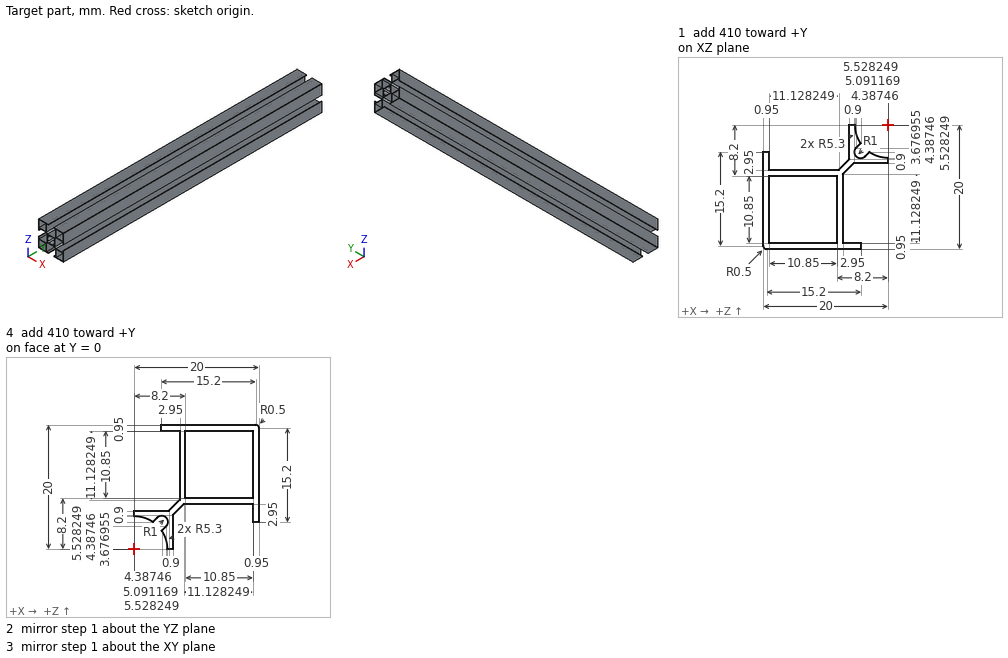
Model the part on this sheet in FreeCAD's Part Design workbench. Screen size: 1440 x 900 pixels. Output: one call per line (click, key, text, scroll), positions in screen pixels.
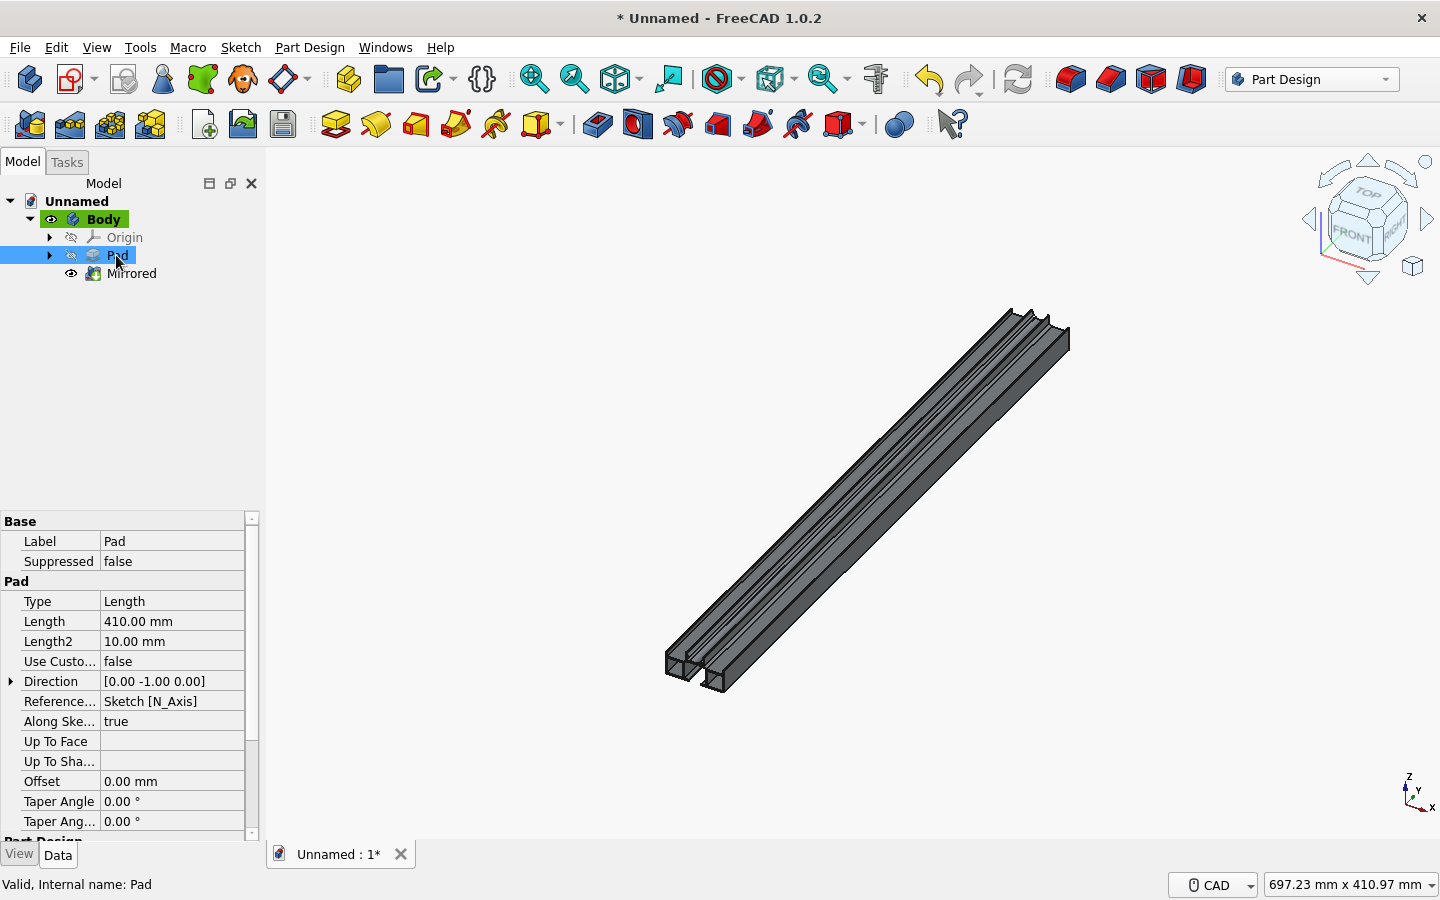
click(30, 124)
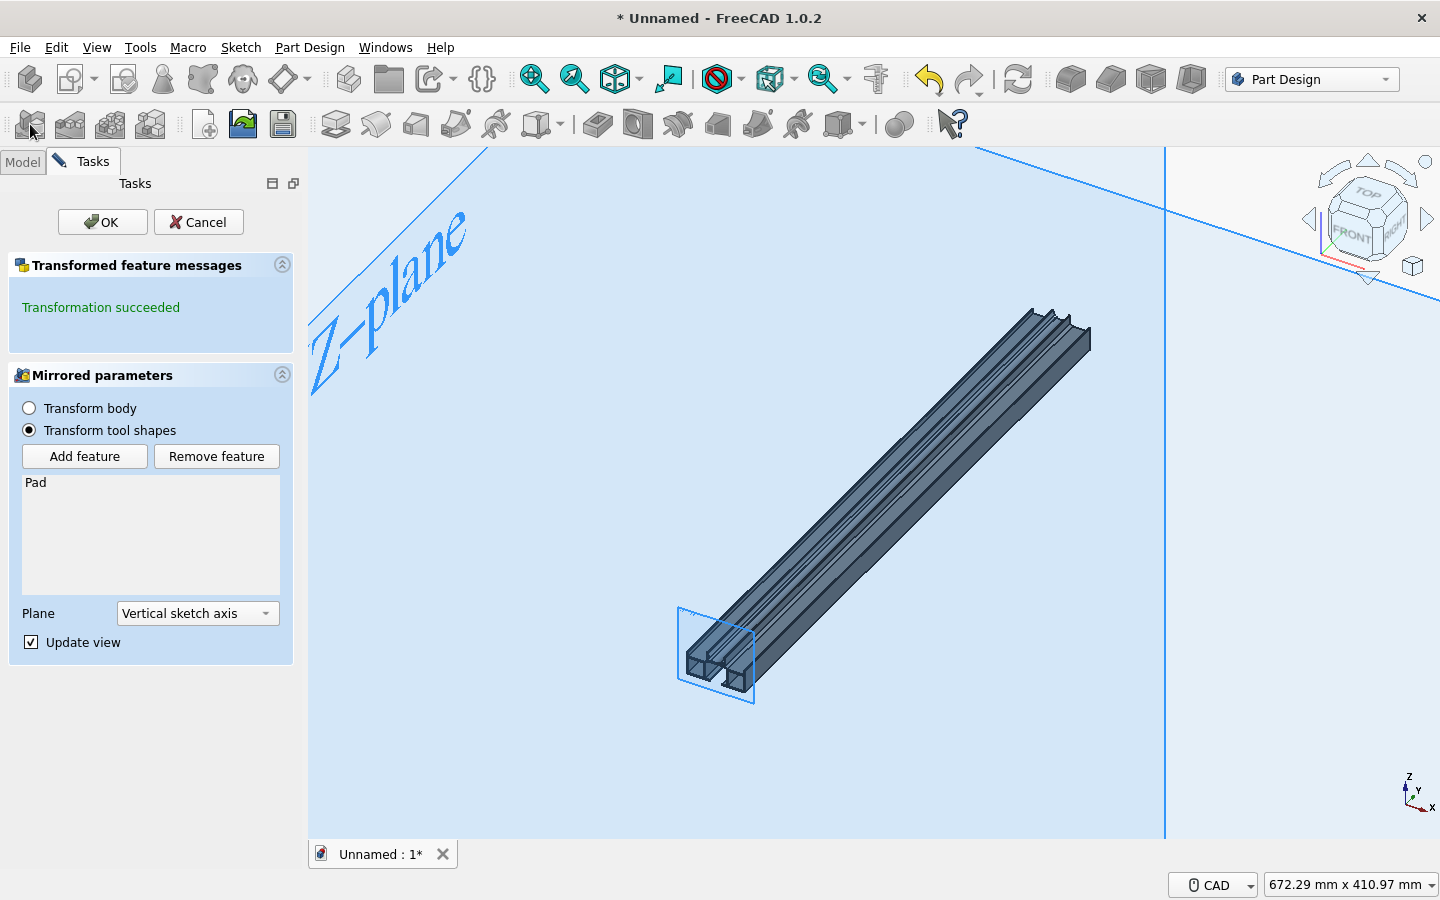
click(198, 614)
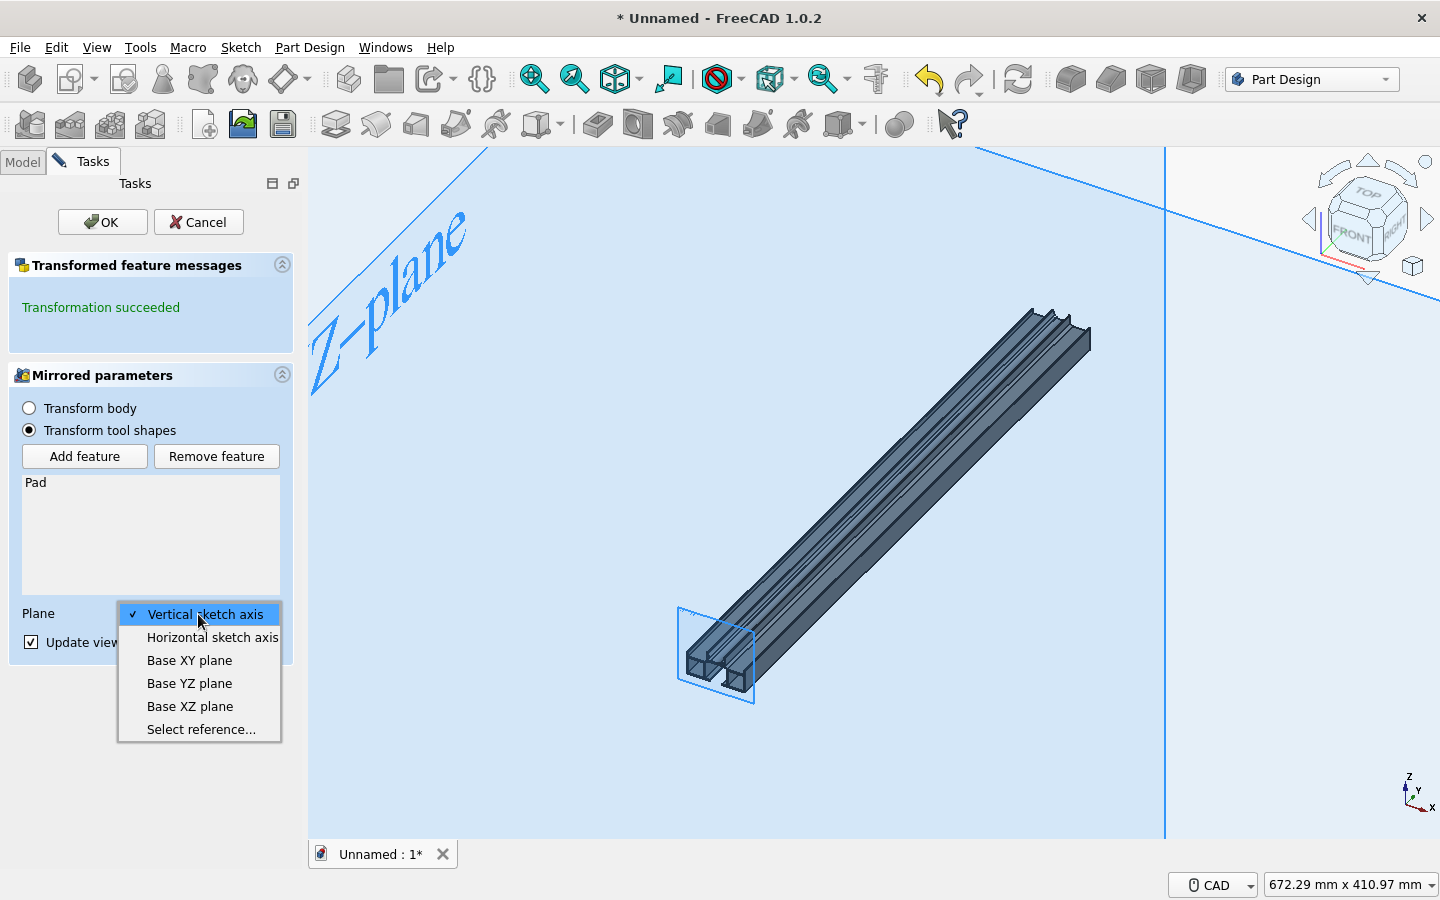
click(198, 660)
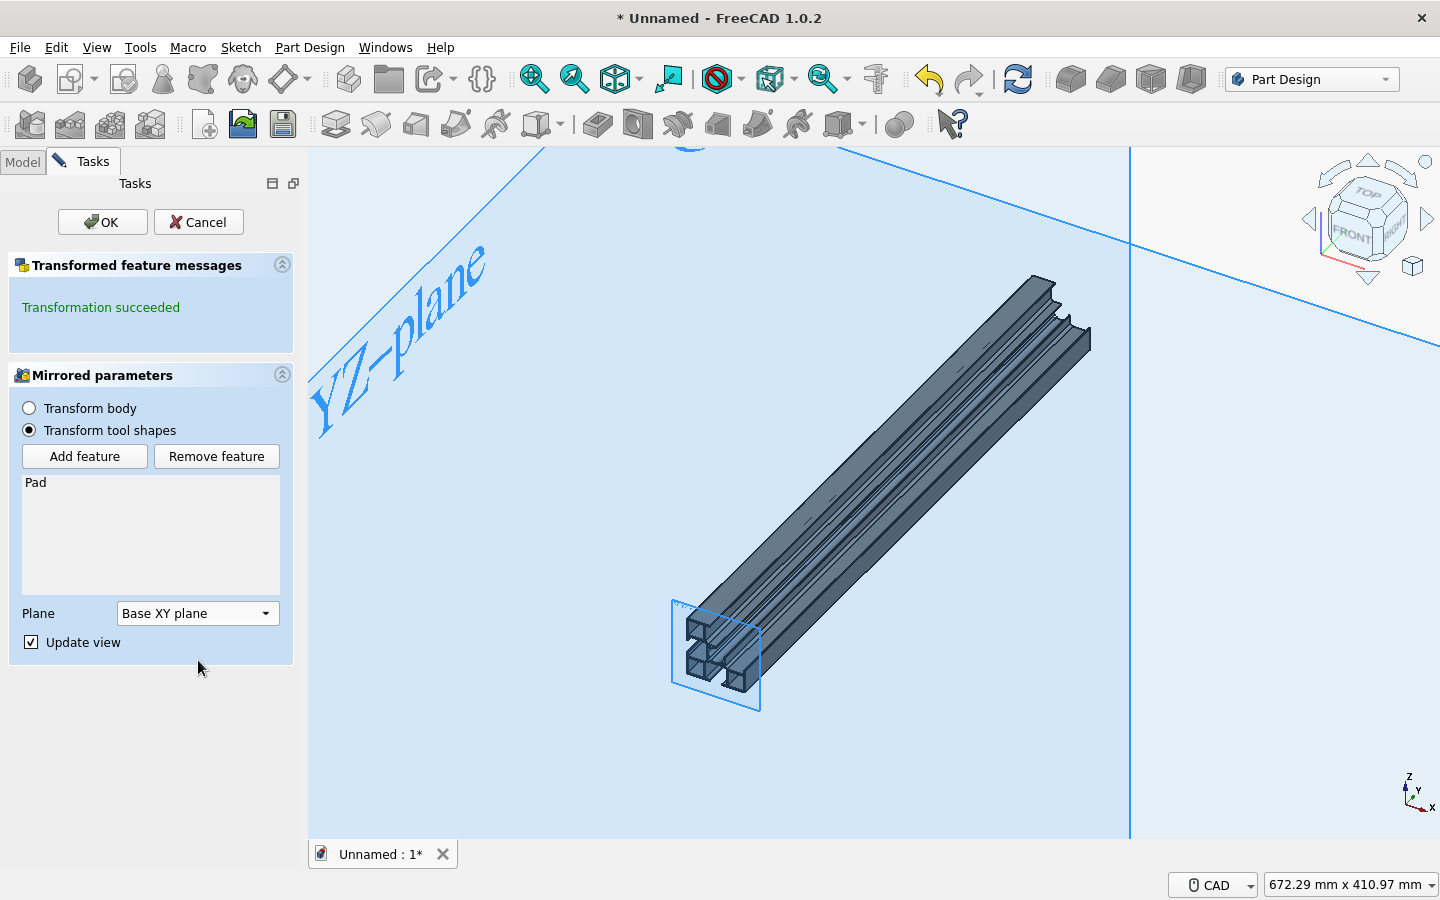
click(103, 222)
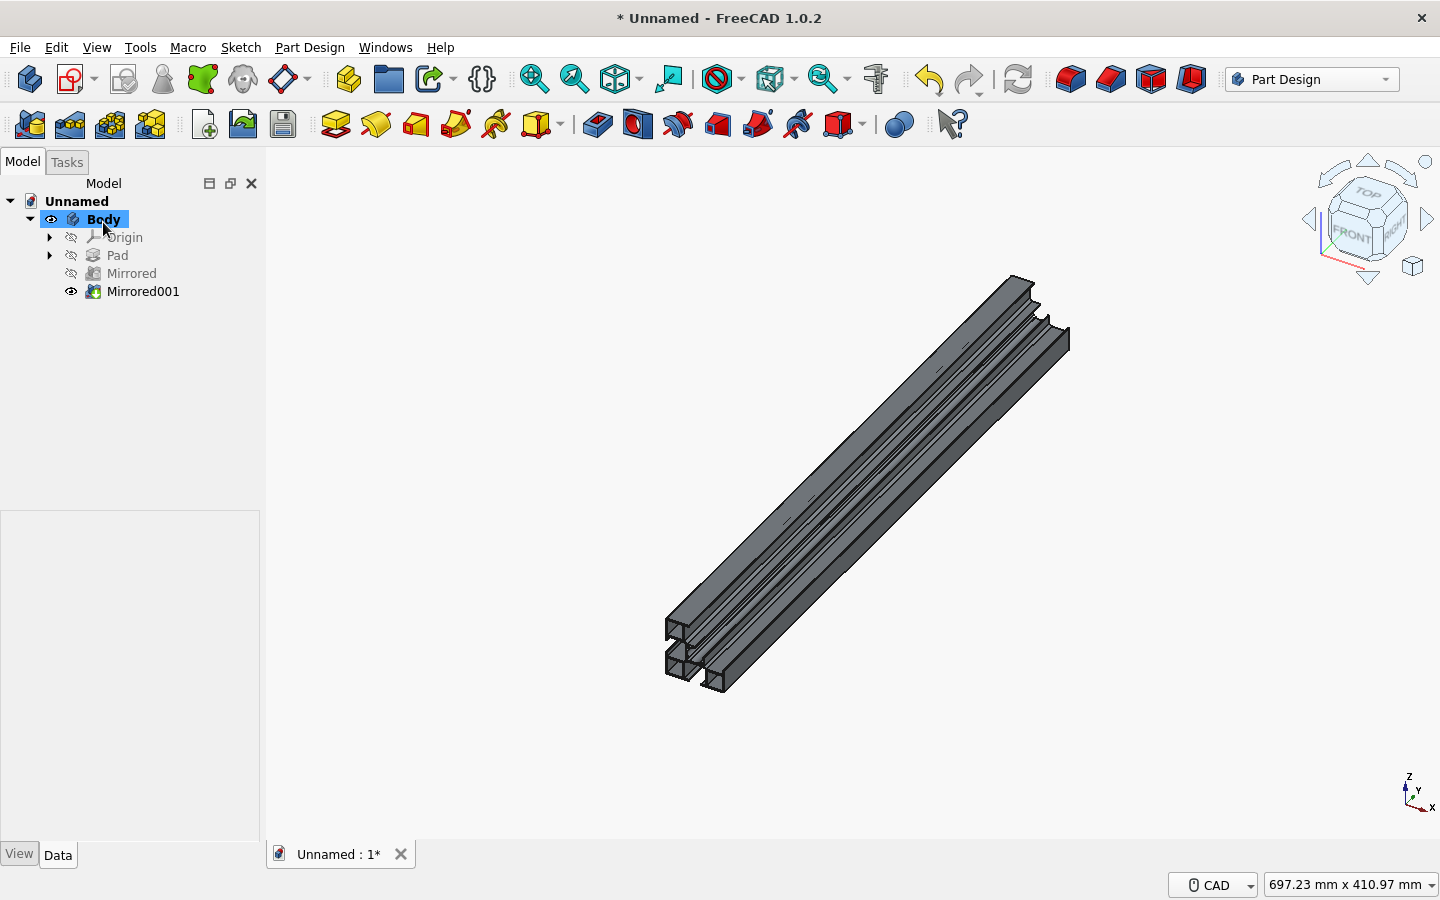
scroll(687, 644, up, 14)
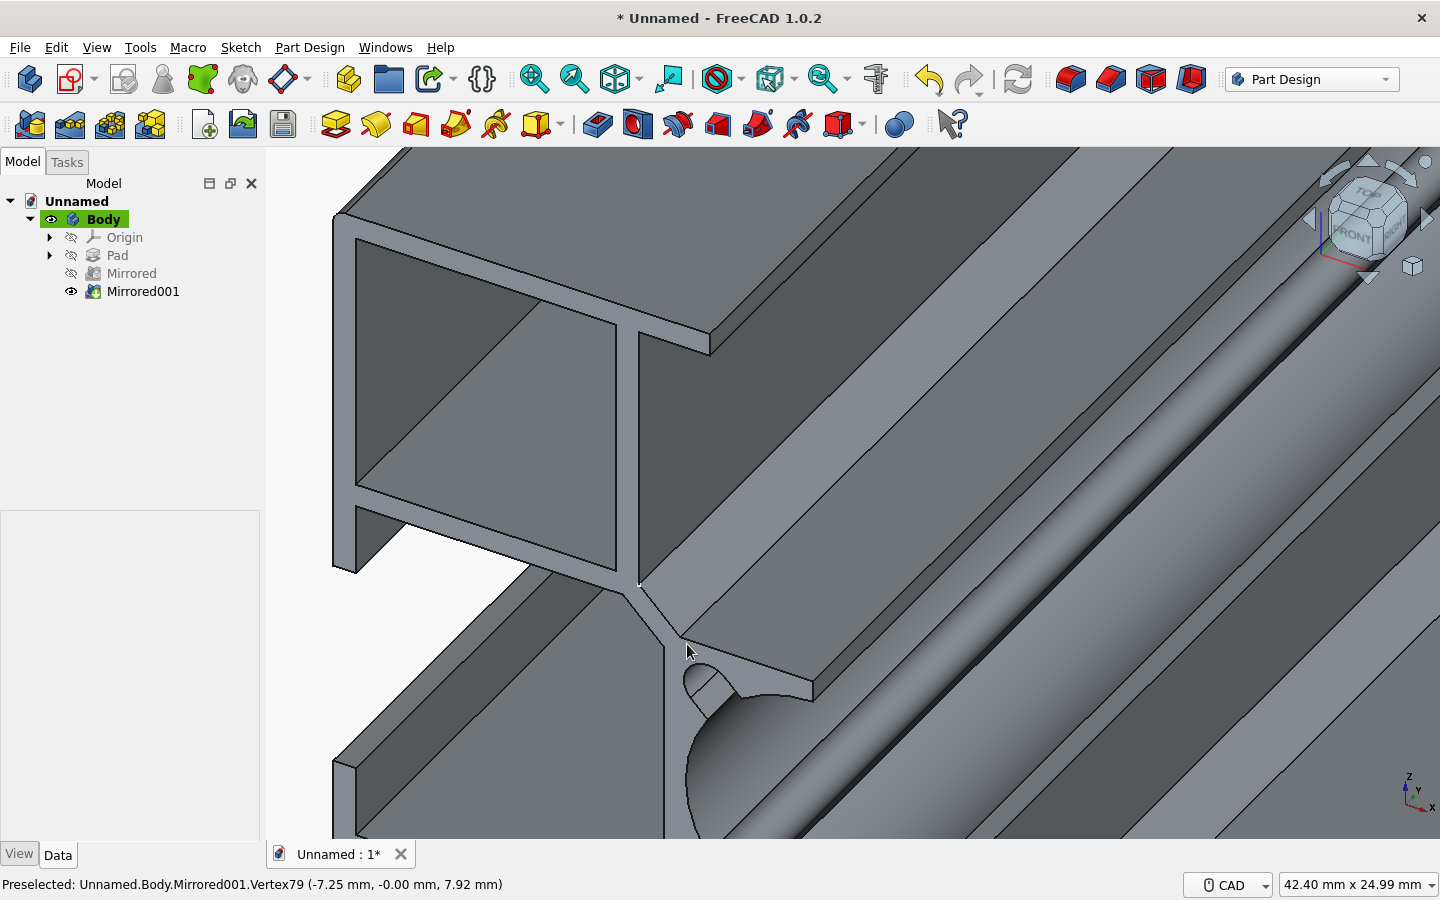
click(676, 646)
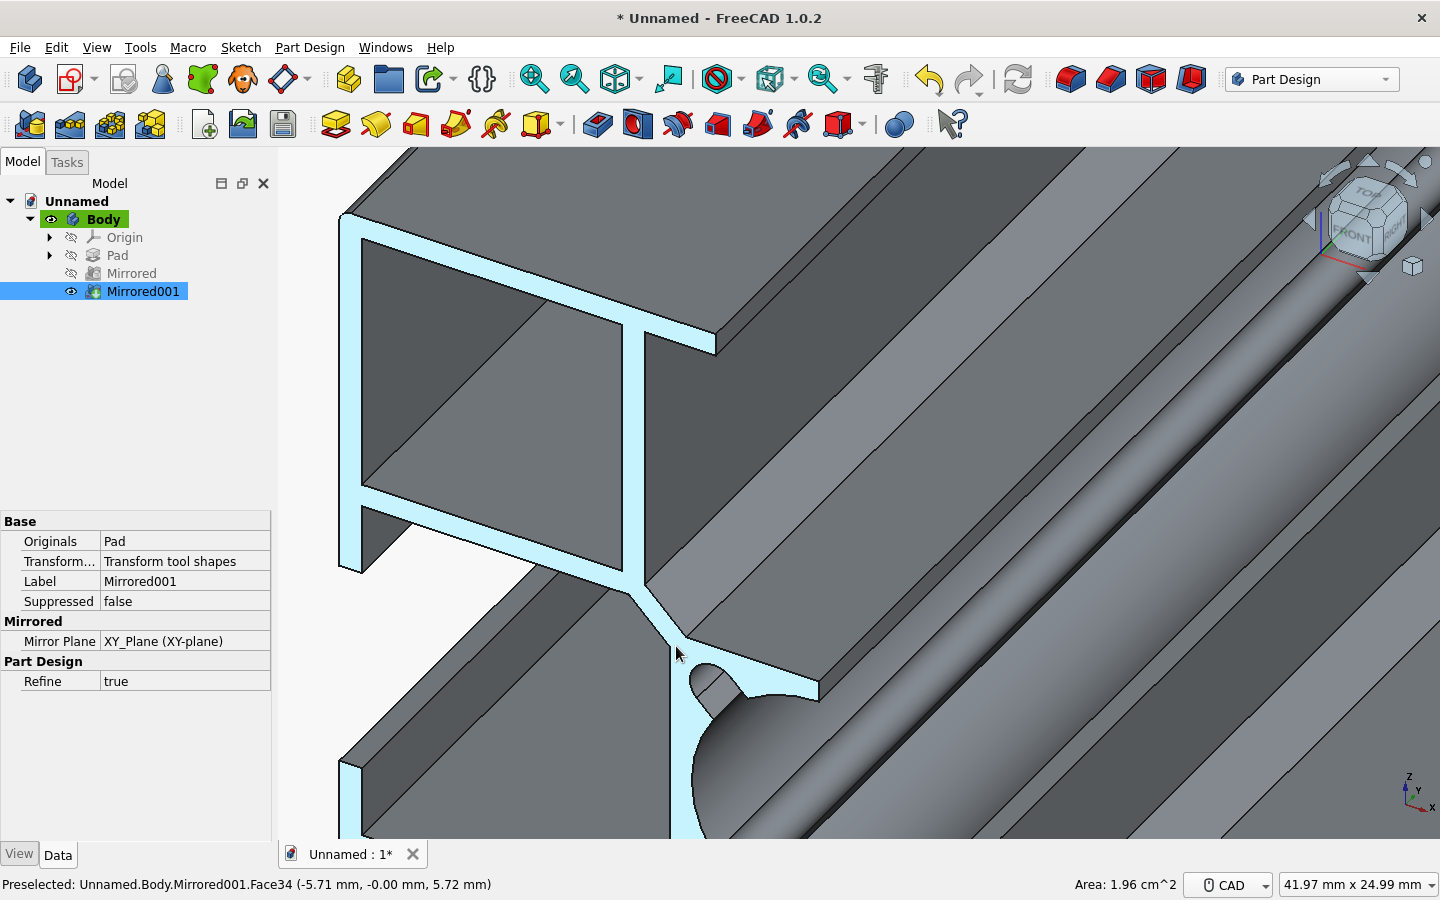
click(70, 80)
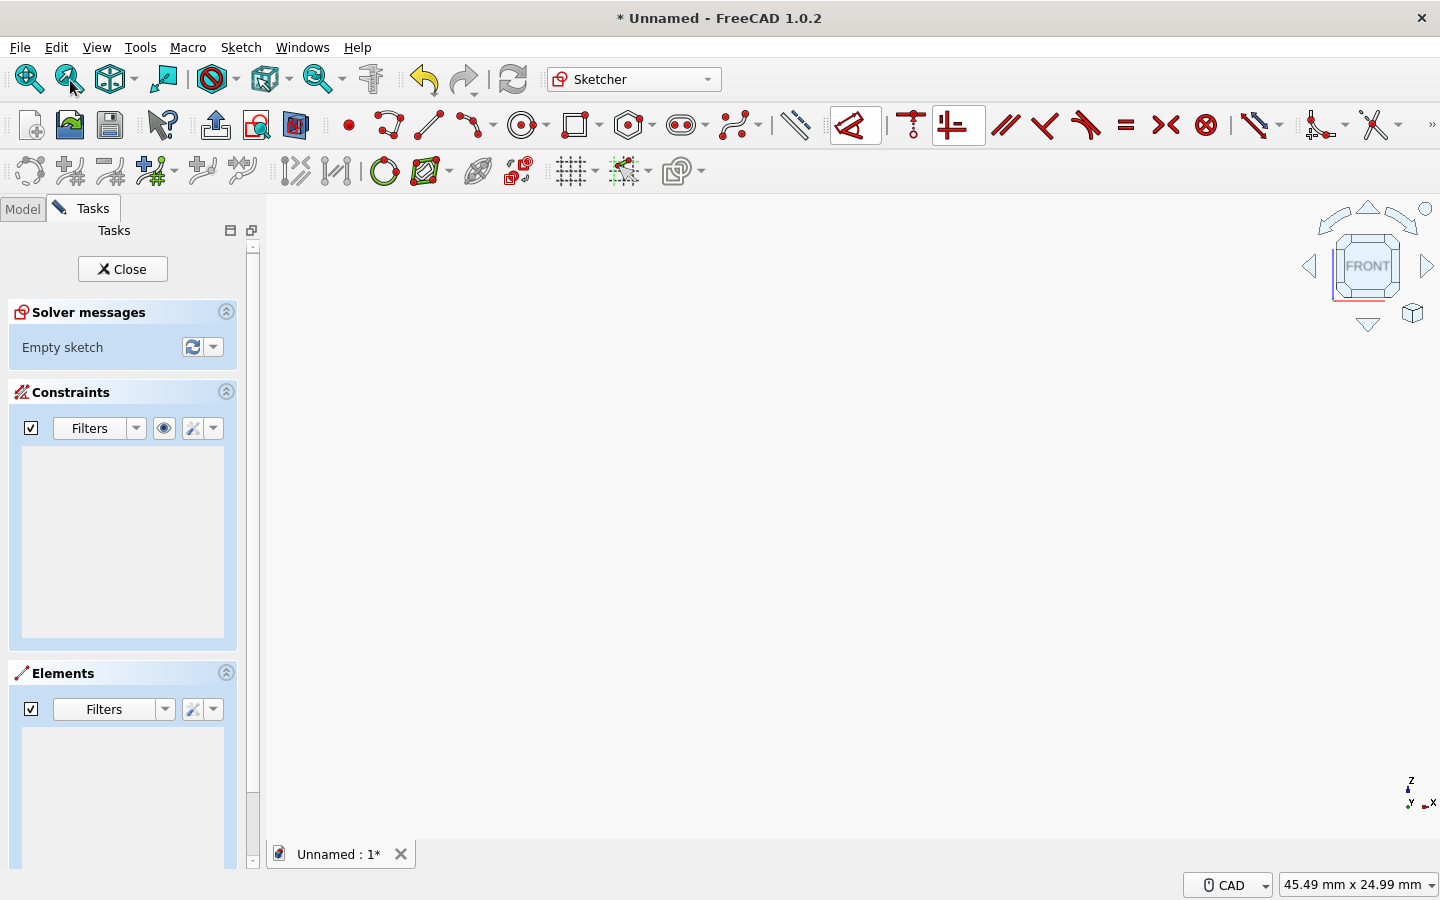
scroll(784, 516, down, 5)